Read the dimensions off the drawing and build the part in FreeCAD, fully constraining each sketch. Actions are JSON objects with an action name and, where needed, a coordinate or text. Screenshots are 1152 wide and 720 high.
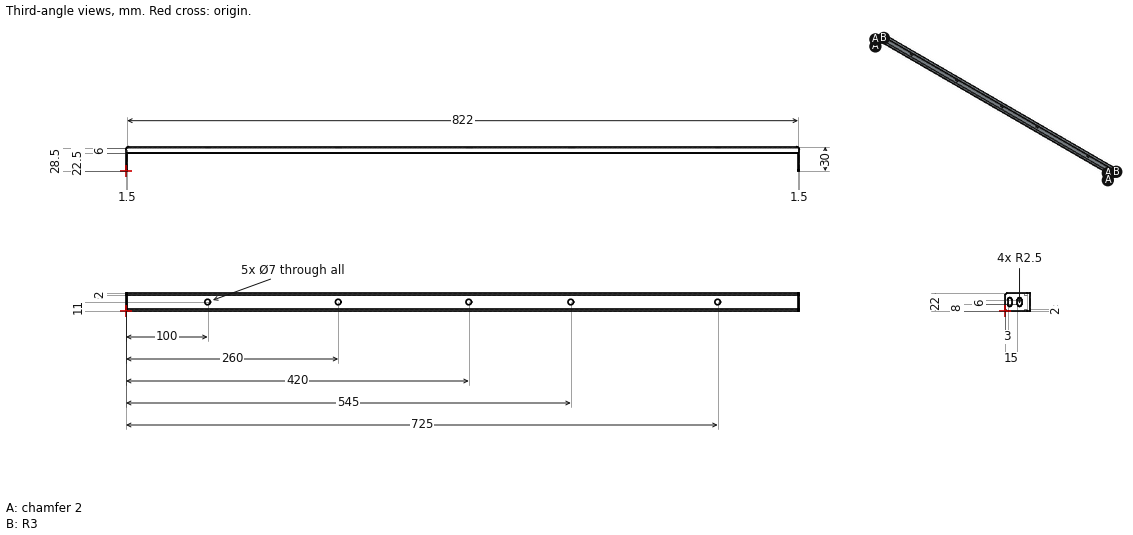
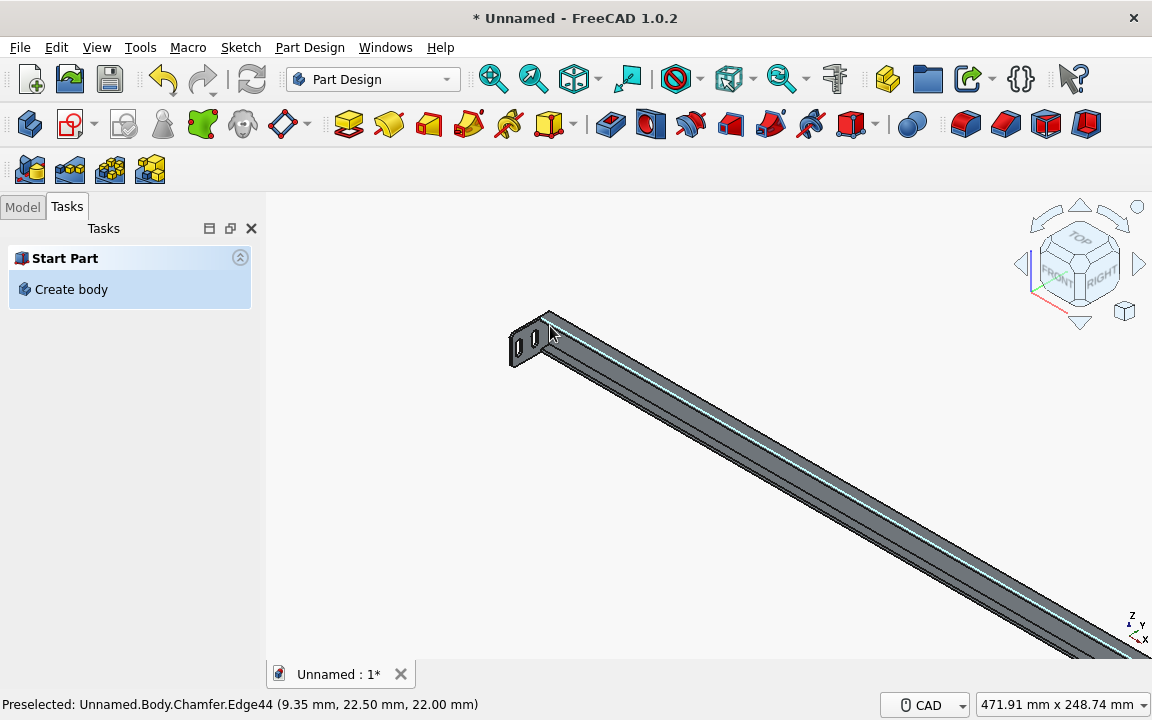
{"action": "left_click", "coordinate": [494, 80]}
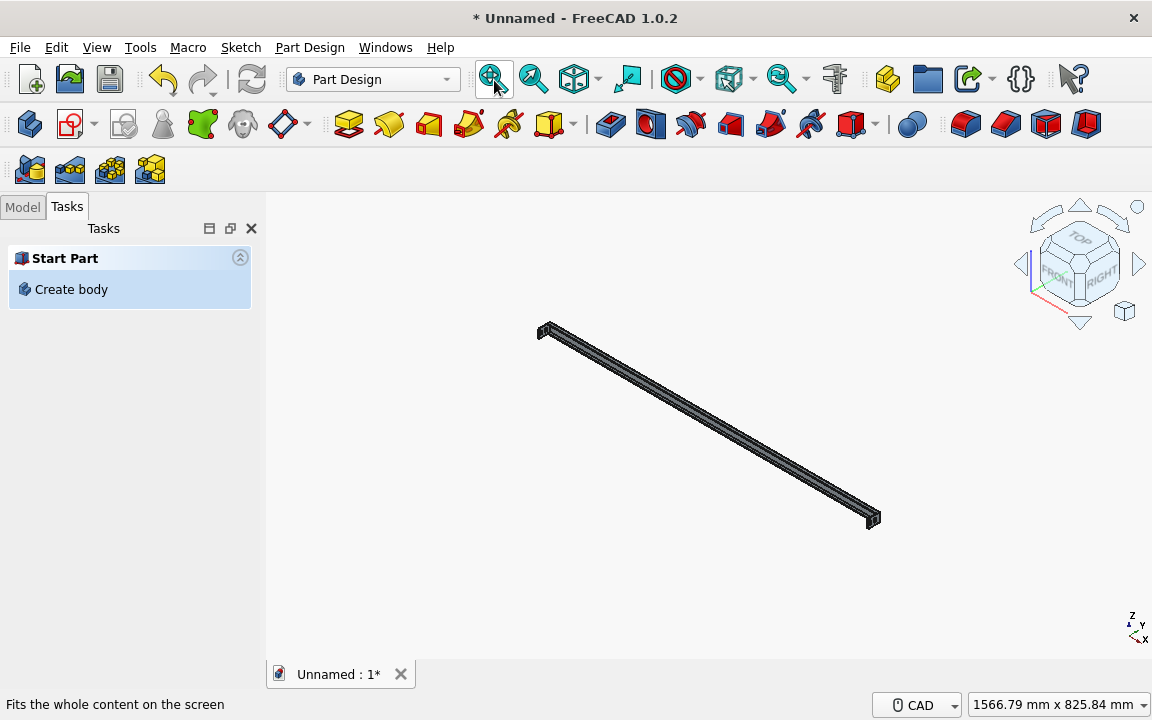
{"action": "key", "text": "2"}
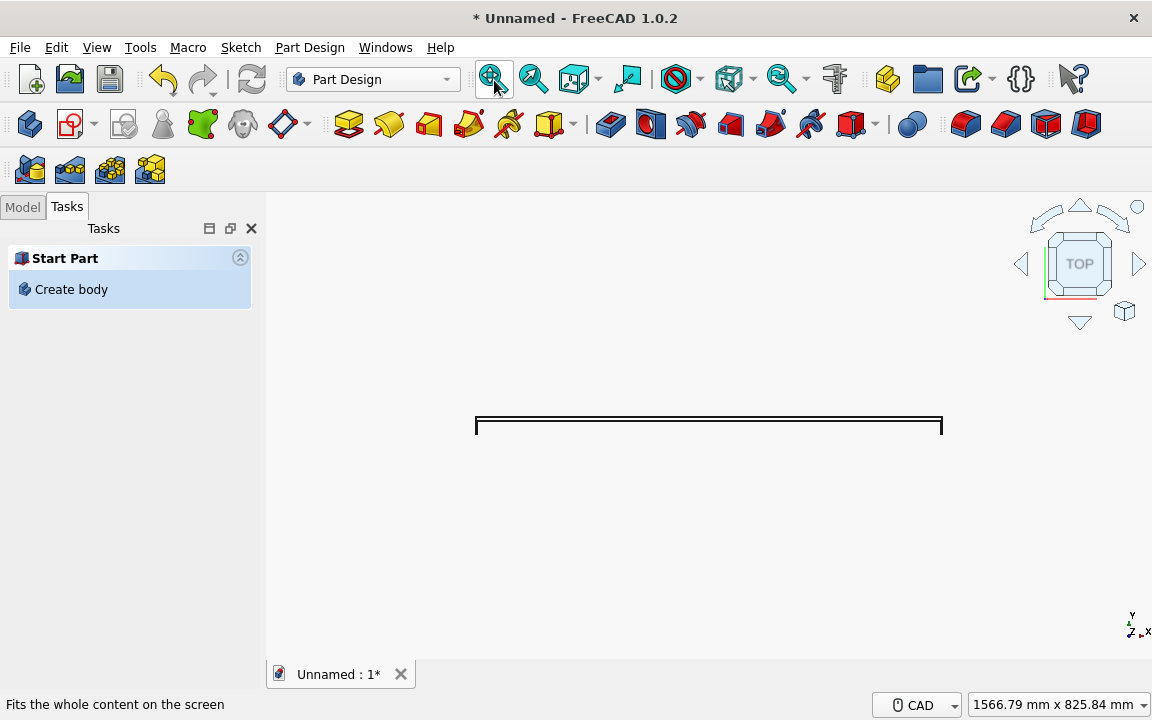
{"action": "scroll", "coordinate": [476, 416], "scroll_direction": "up", "scroll_amount": 6}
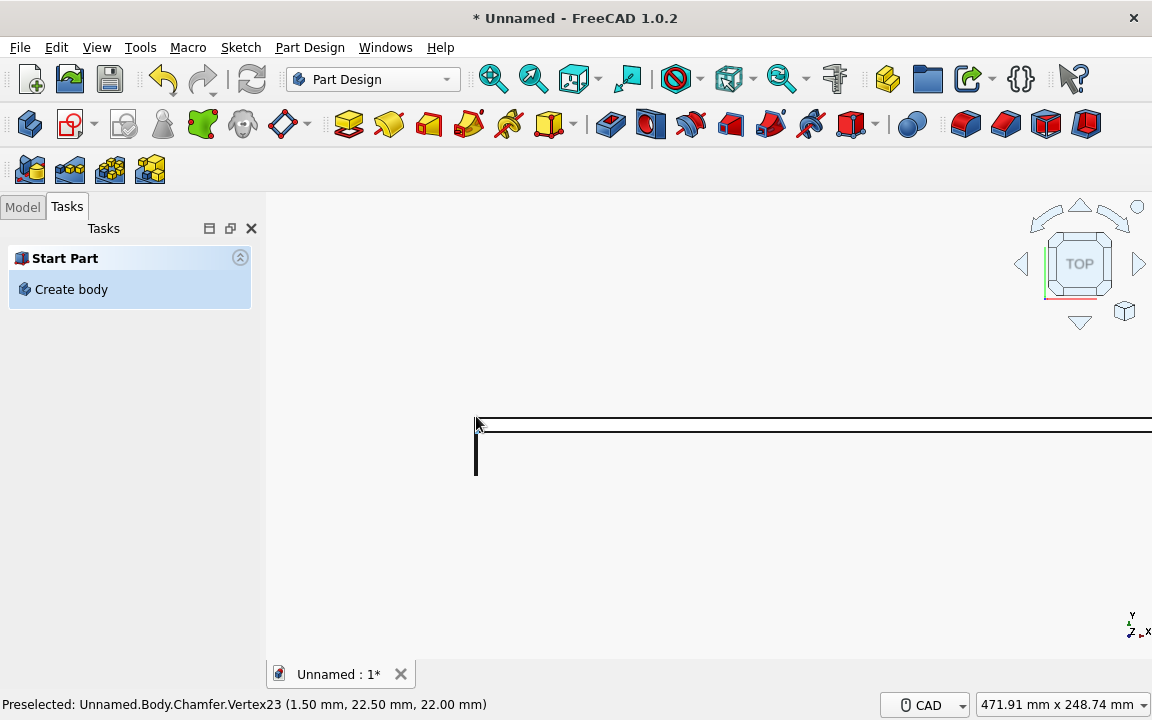
{"action": "left_click", "coordinate": [494, 80]}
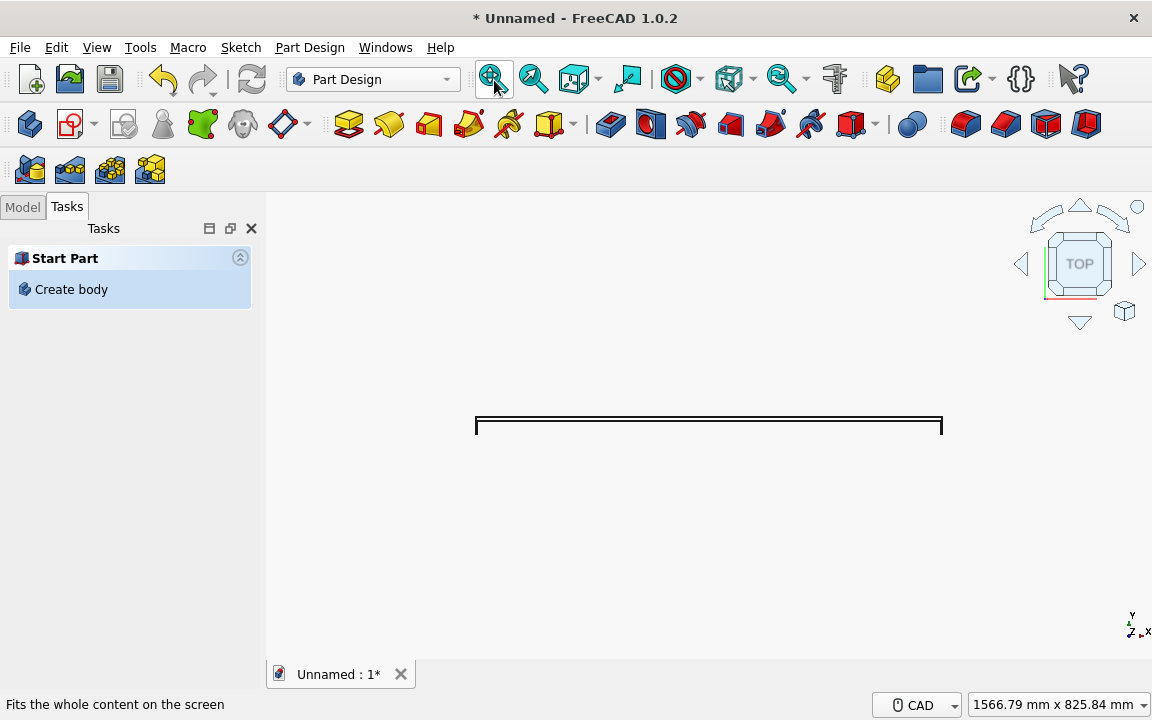
{"action": "key", "text": "0"}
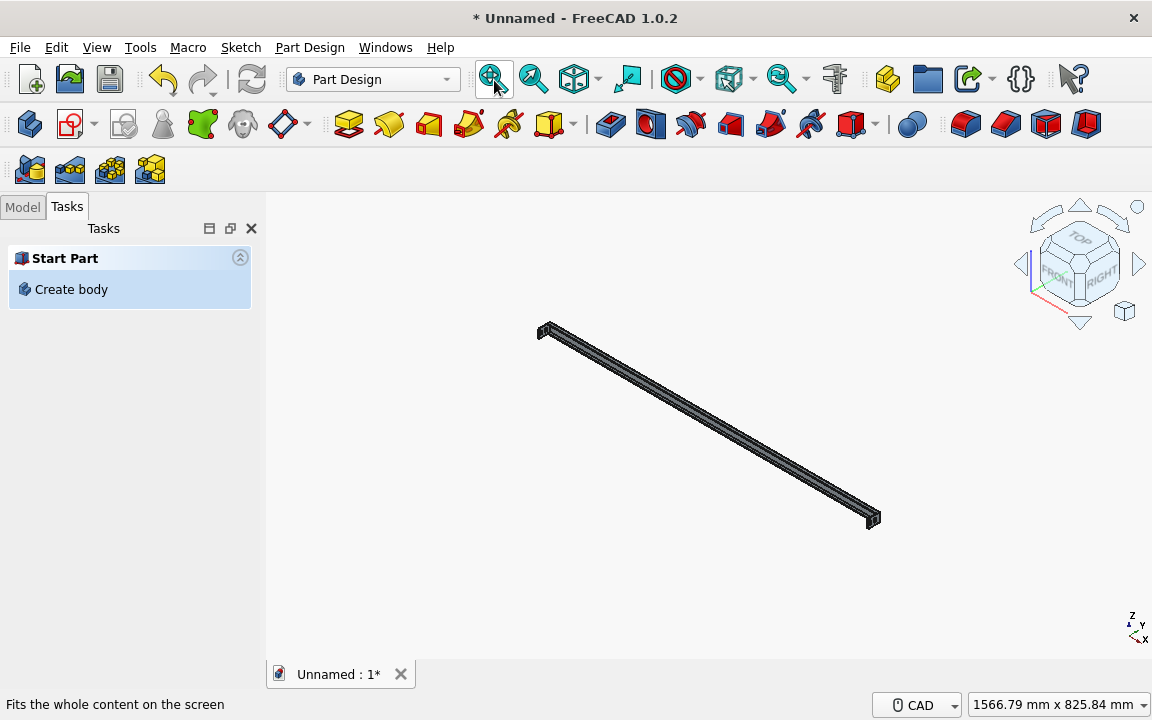
{"action": "left_click", "coordinate": [494, 80]}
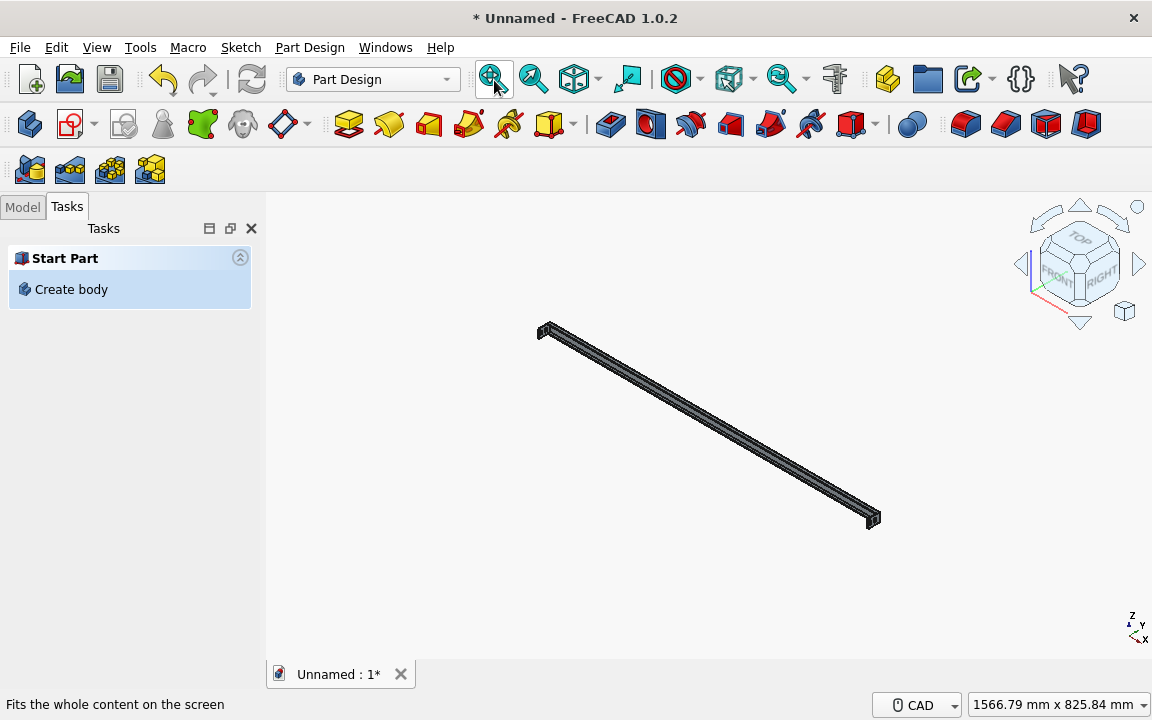
{"action": "scroll", "coordinate": [550, 326], "scroll_direction": "up", "scroll_amount": 6}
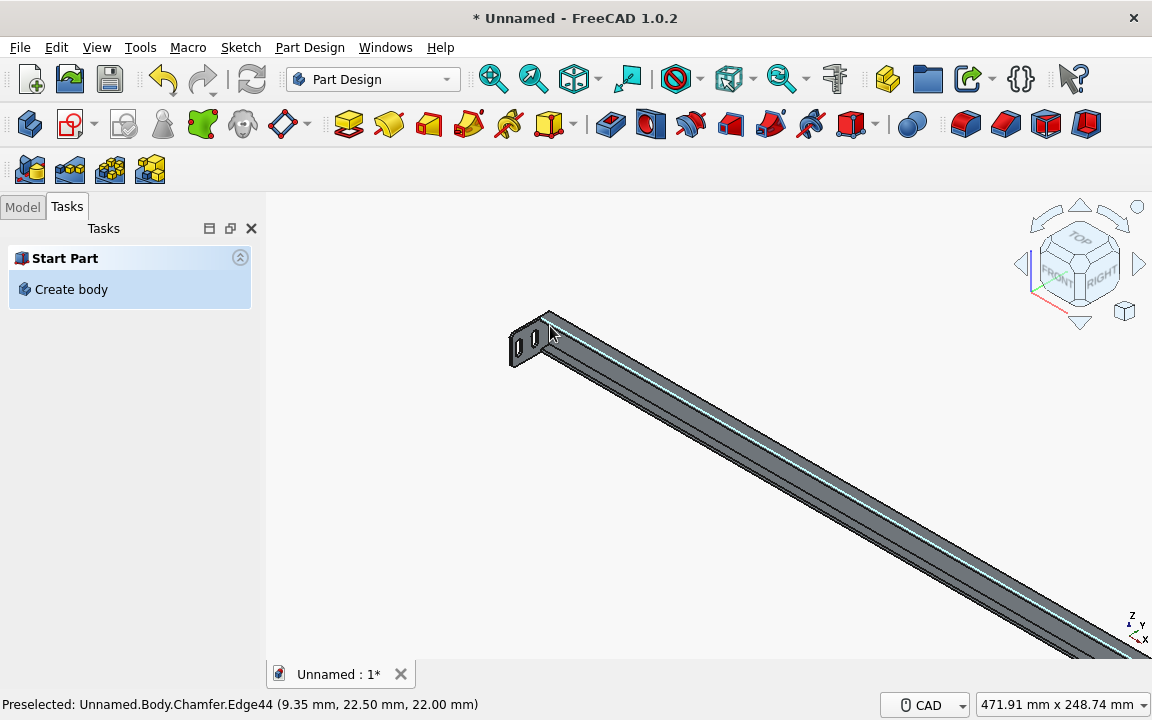
{"action": "left_click", "coordinate": [494, 80]}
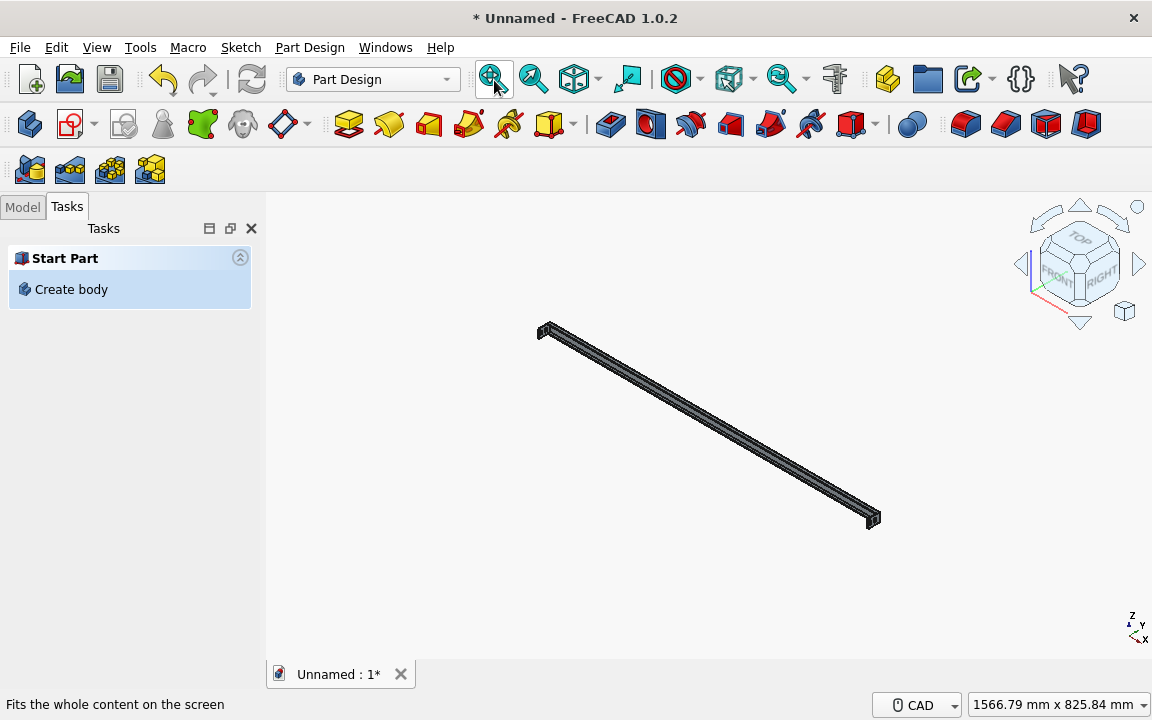
{"action": "key", "text": "1"}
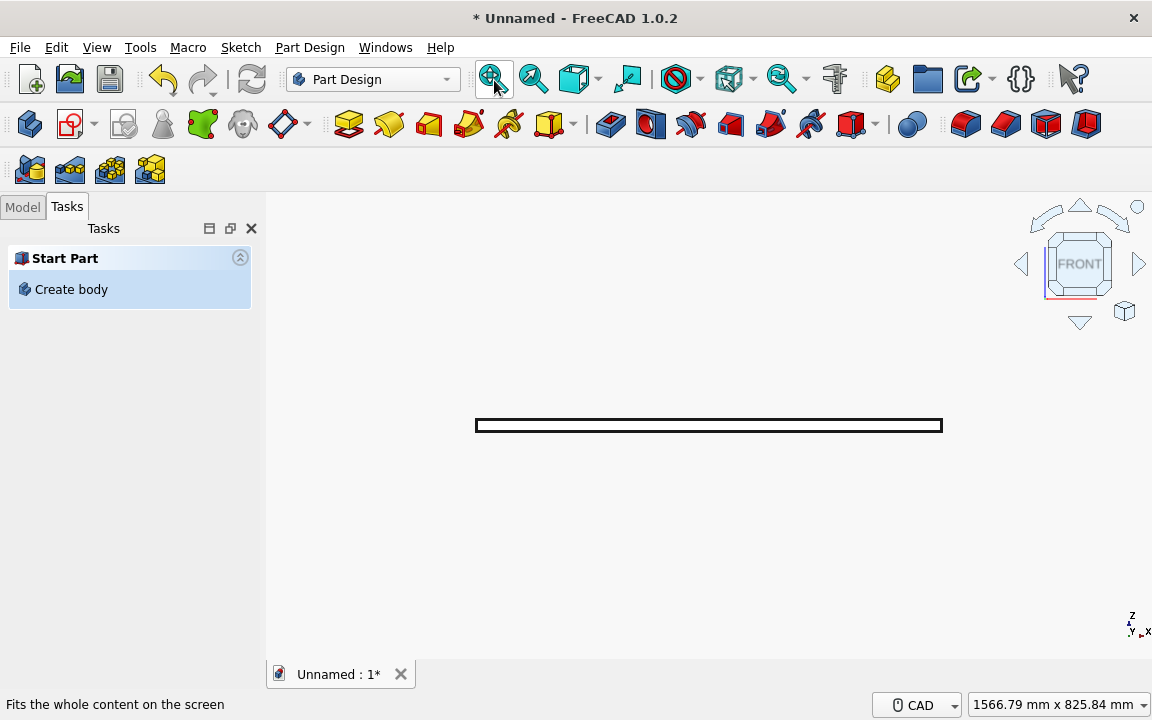
{"action": "scroll", "coordinate": [476, 424], "scroll_direction": "up", "scroll_amount": 6}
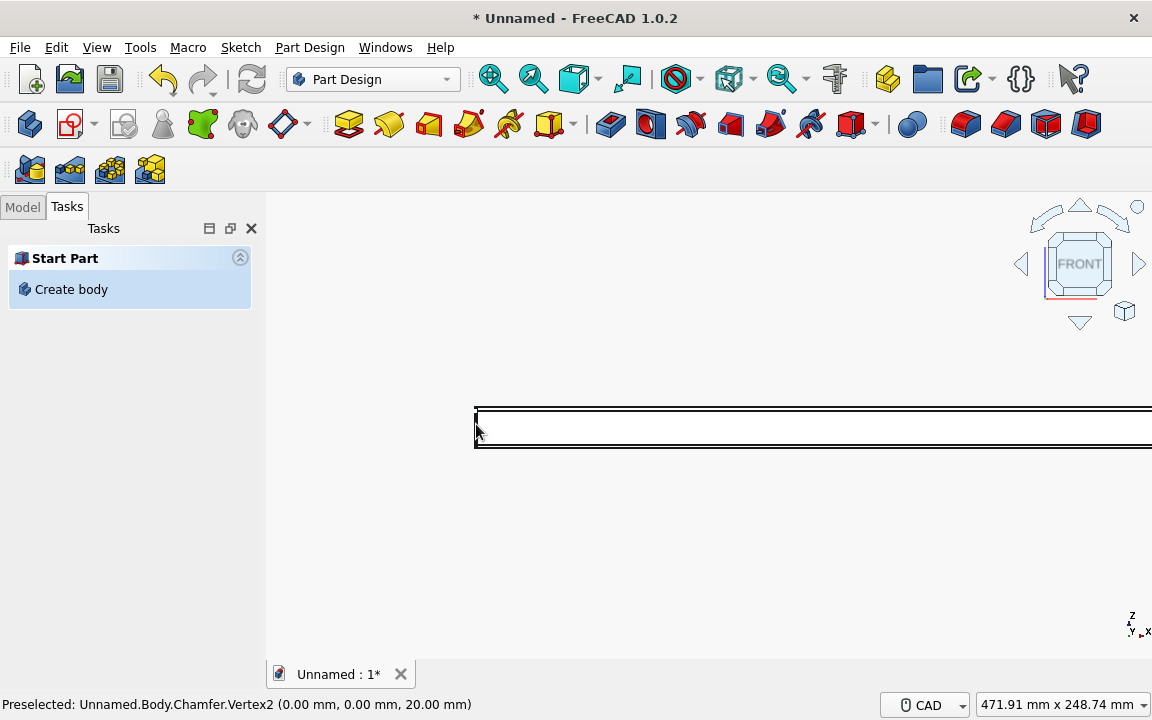
{"action": "left_click", "coordinate": [494, 80]}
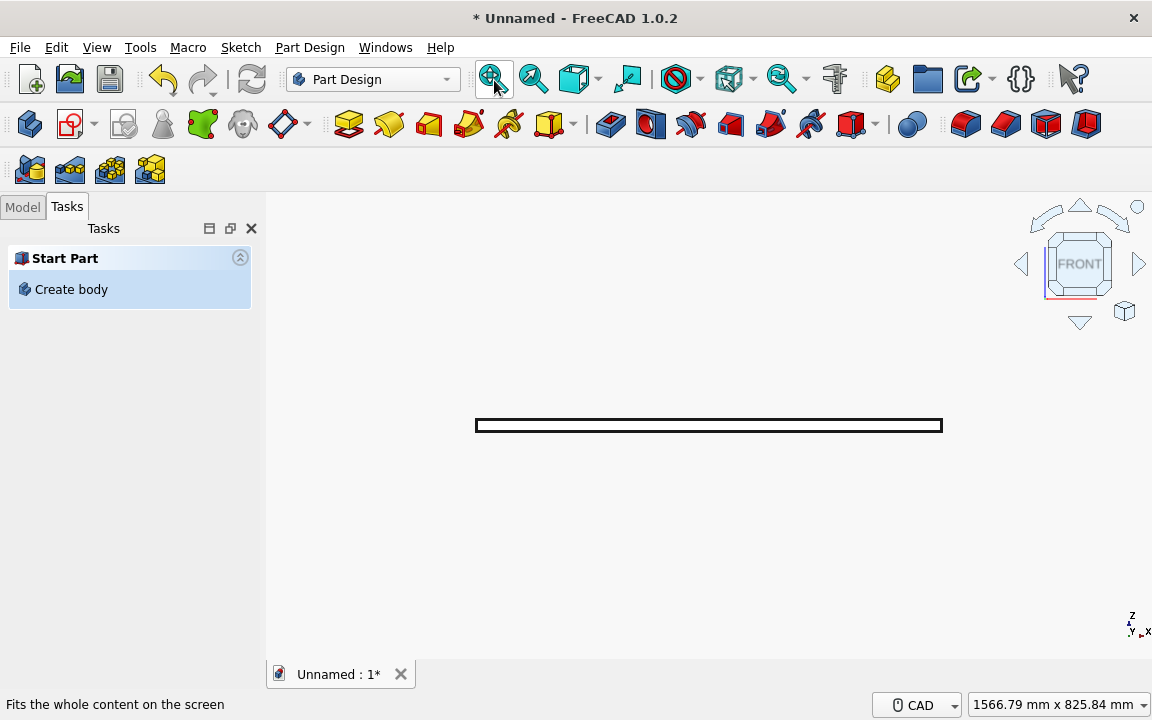
{"action": "key", "text": "3"}